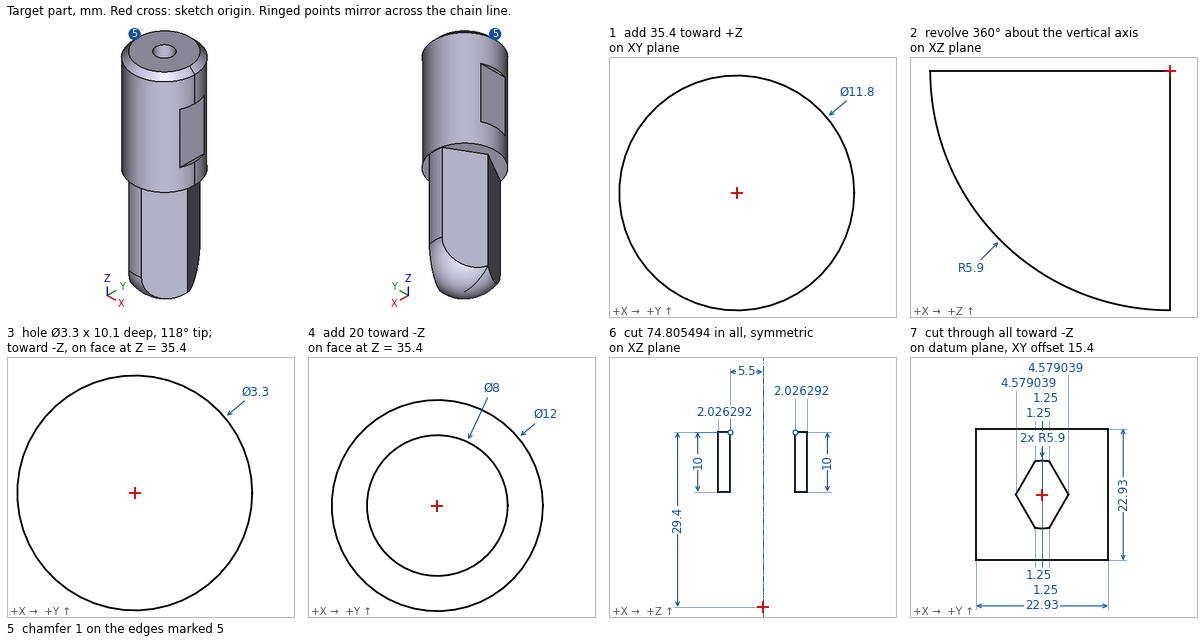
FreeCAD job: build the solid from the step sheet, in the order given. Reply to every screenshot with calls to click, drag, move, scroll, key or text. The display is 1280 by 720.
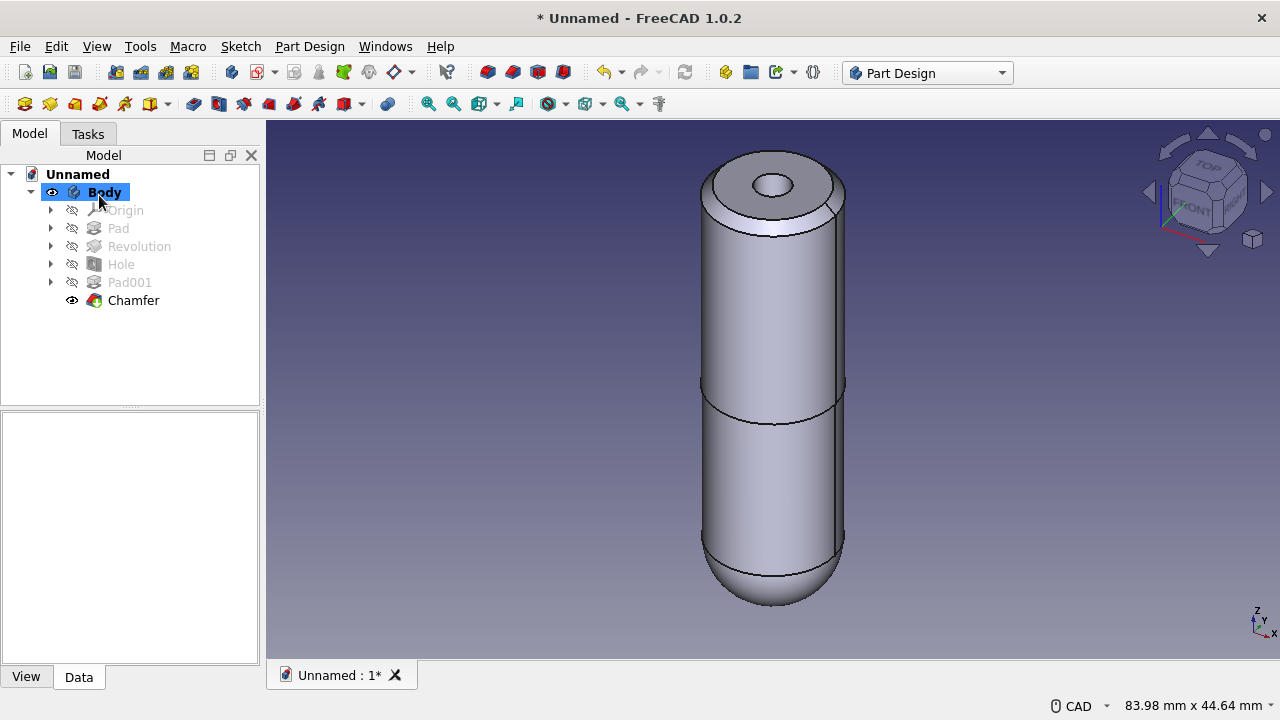
click(256, 72)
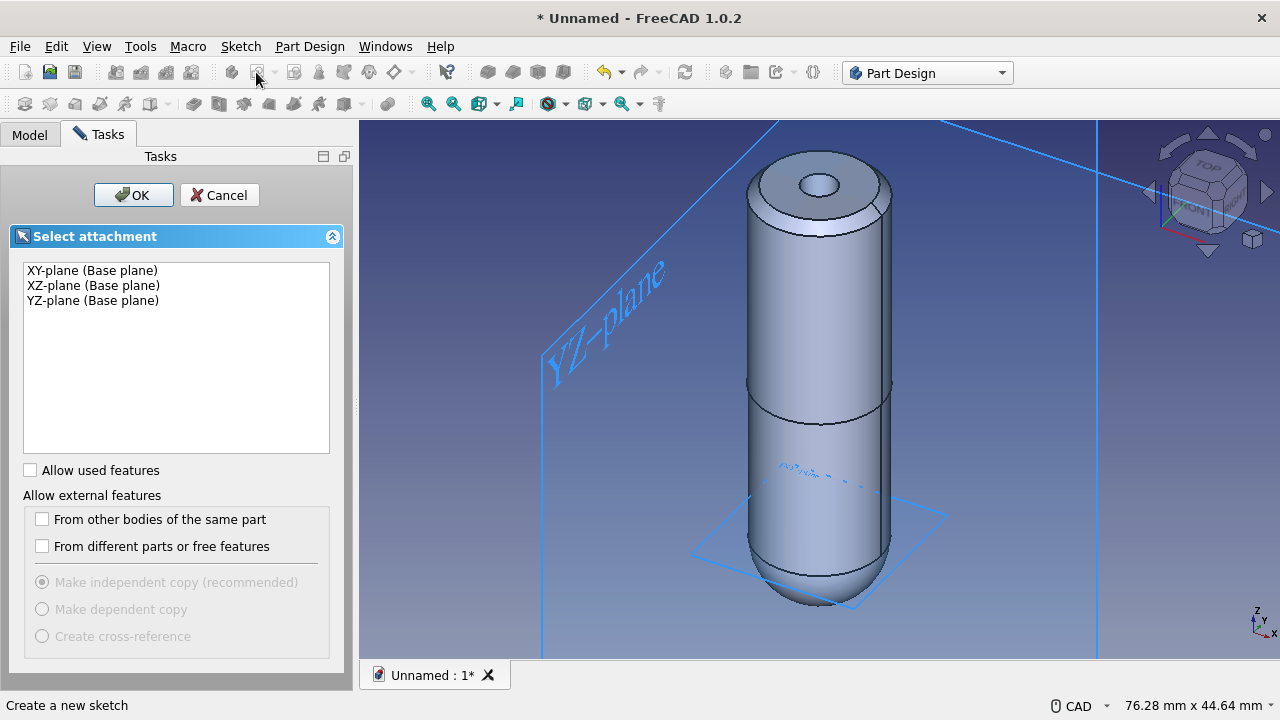
click(84, 286)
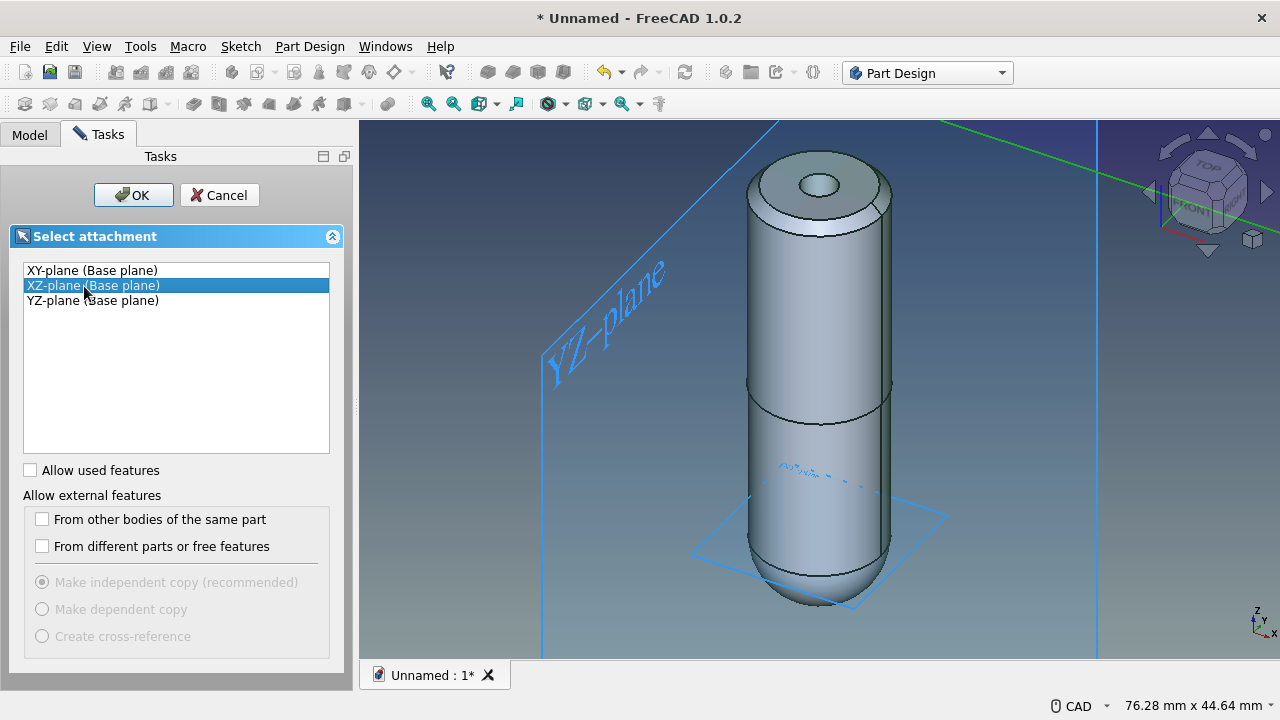
click(134, 195)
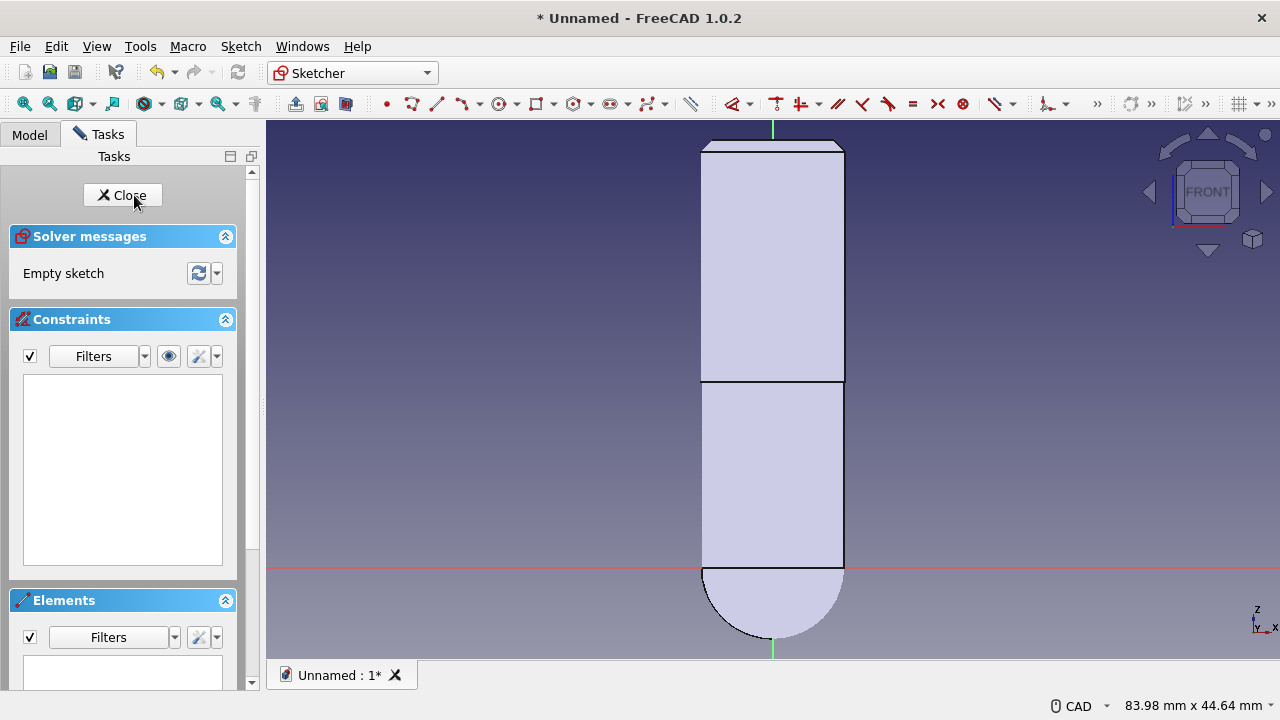
click(346, 104)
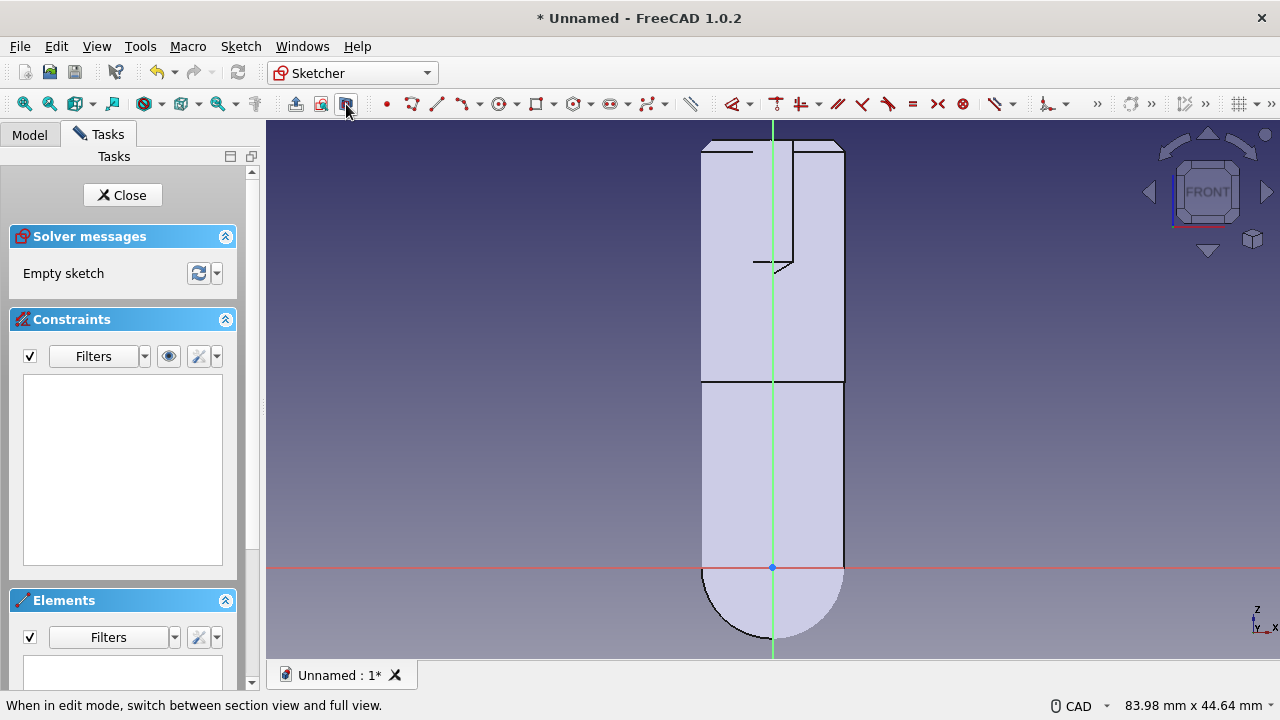
key(g)
key(r)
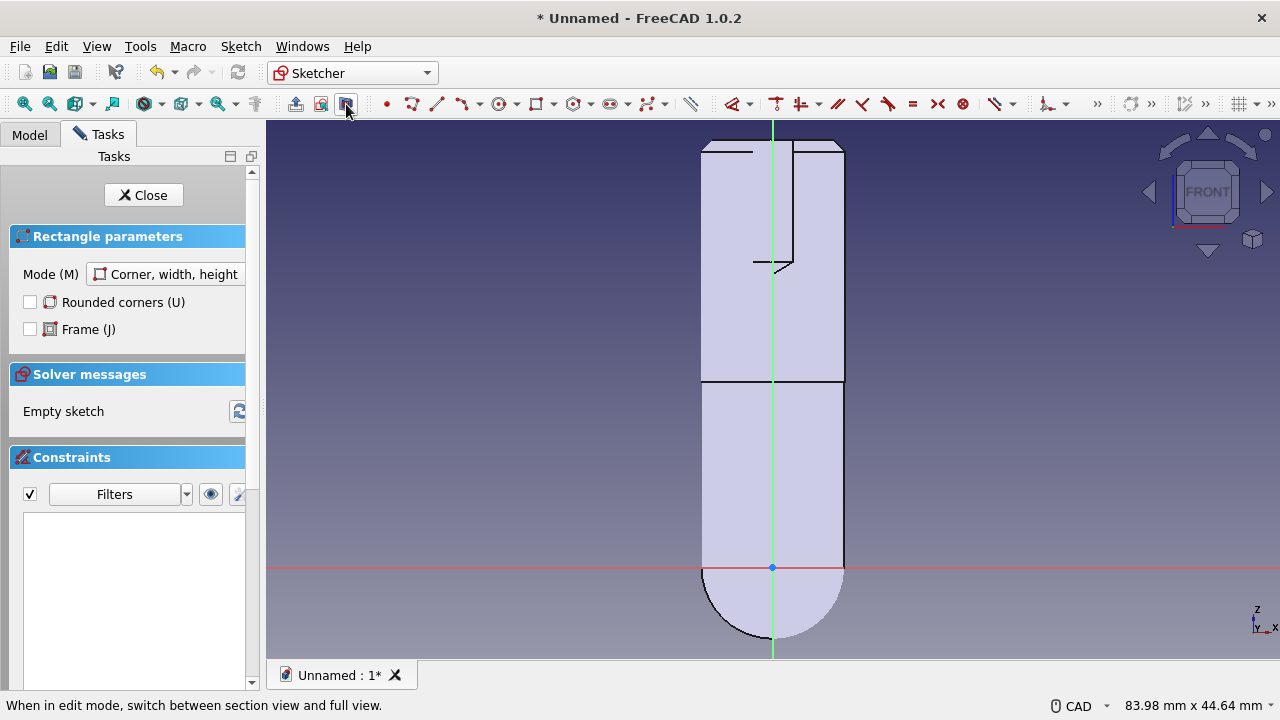
click(682, 213)
move(706, 333)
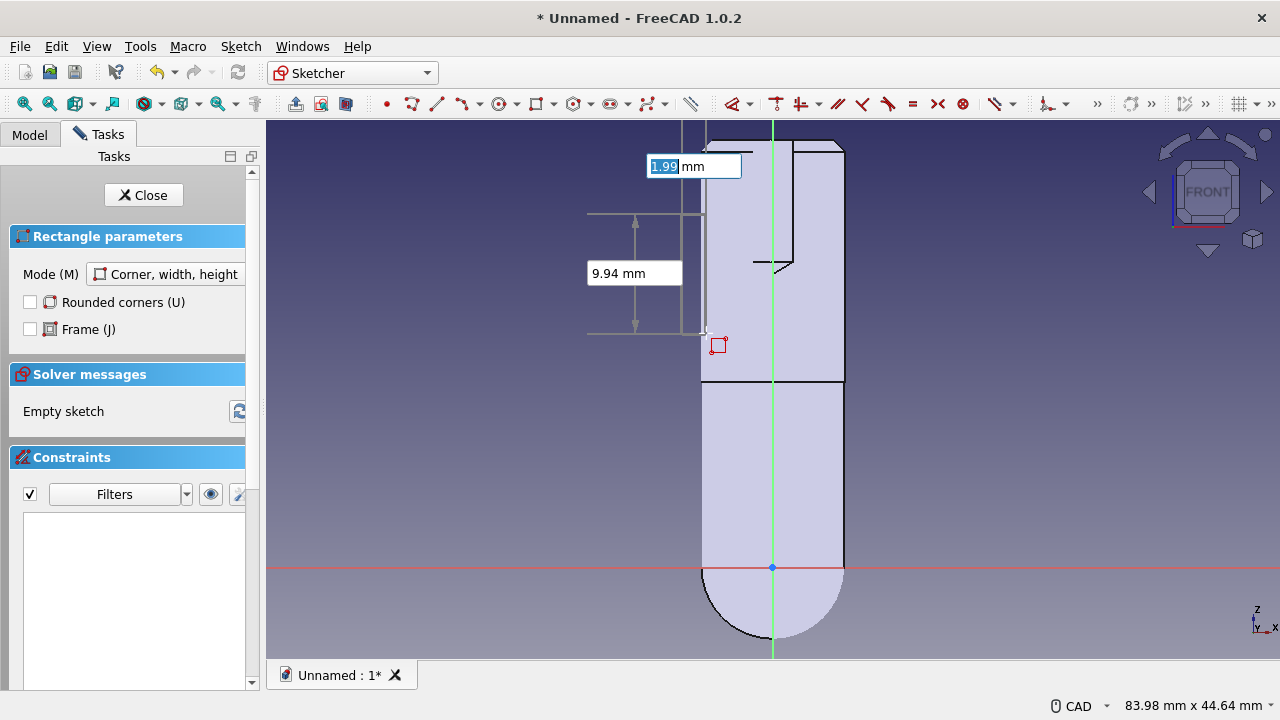
text(2.026292)
key(Tab)
text(10)
key(Return)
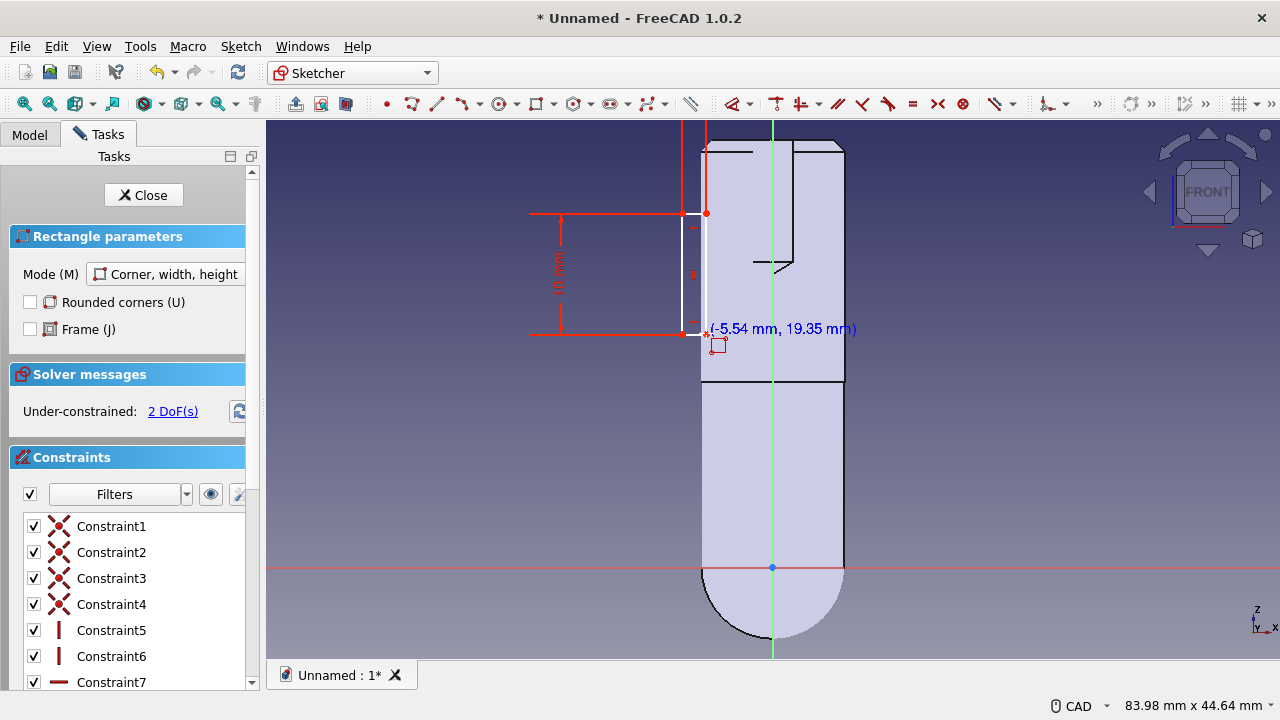
click(839, 213)
move(864, 333)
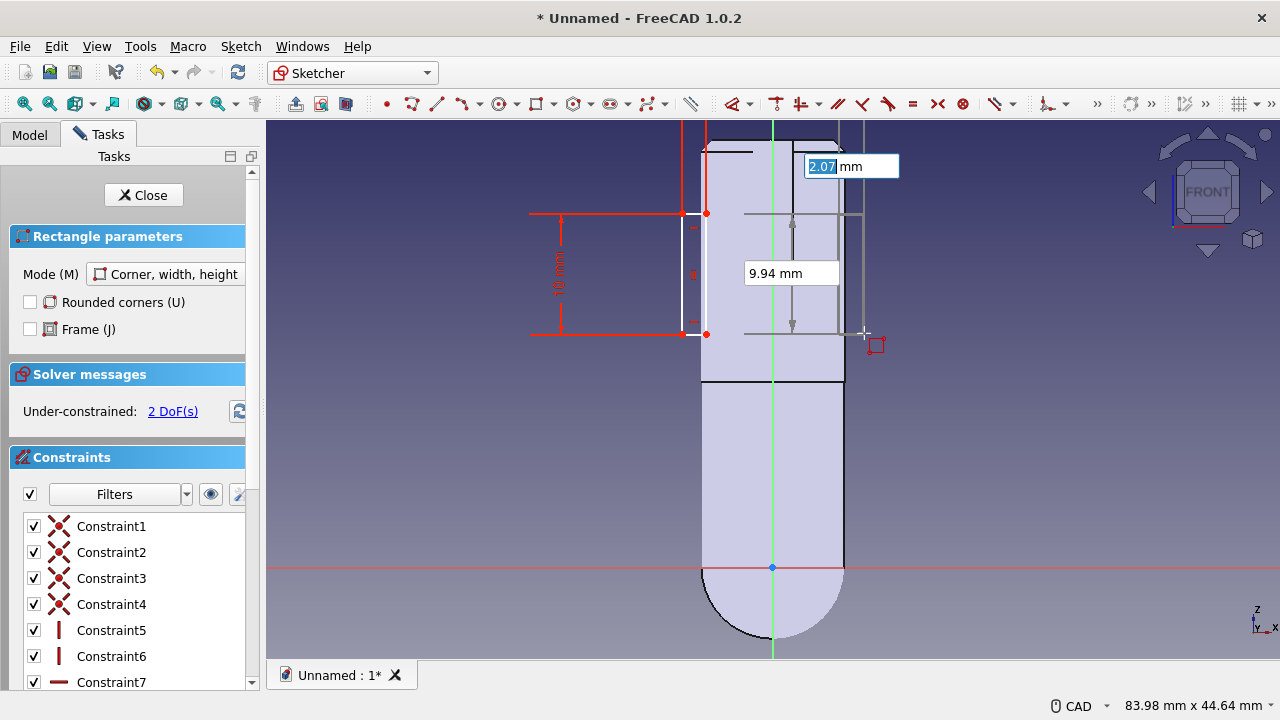
text(2.026292)
key(Tab)
text(10)
key(Return)
key(Escape)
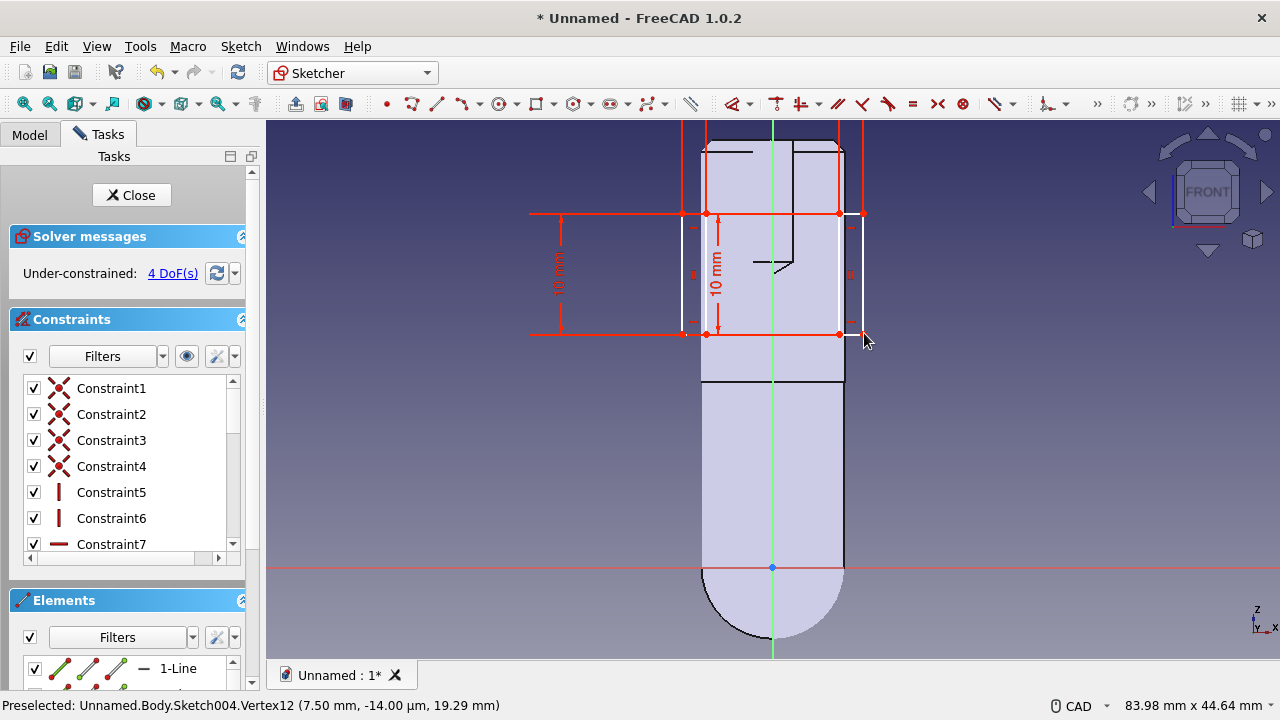
click(706, 214)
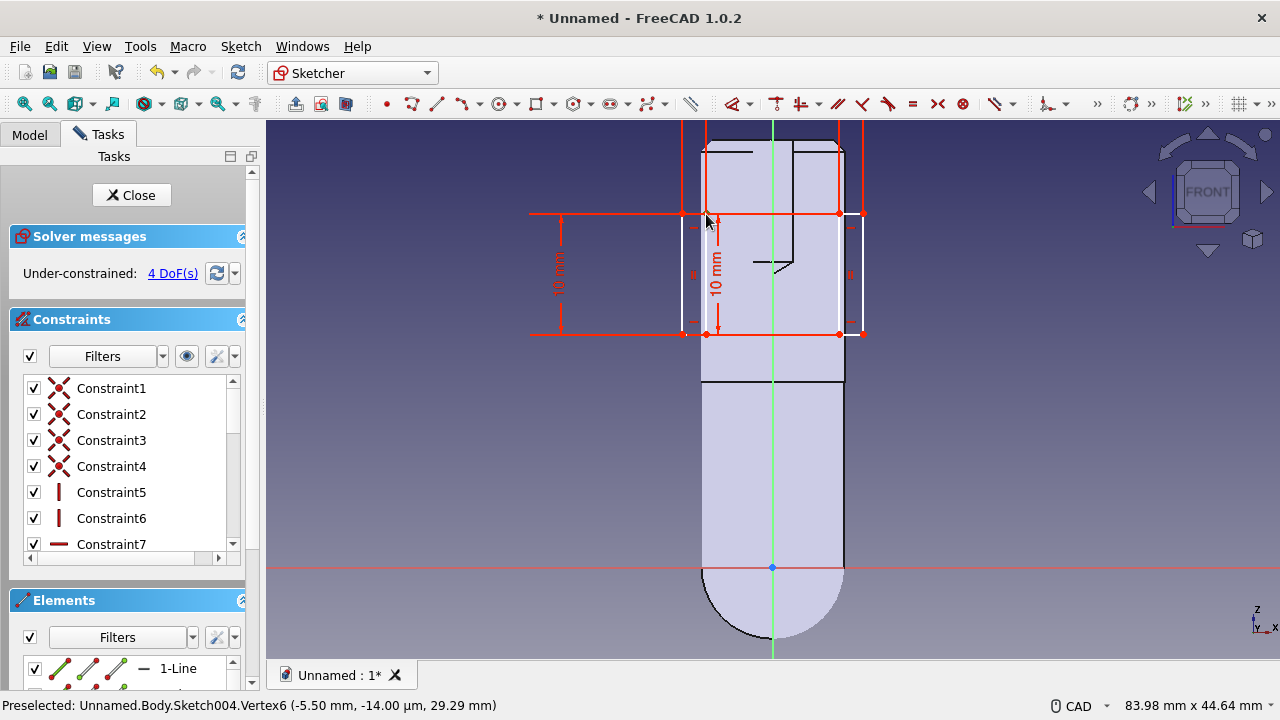
click(839, 214)